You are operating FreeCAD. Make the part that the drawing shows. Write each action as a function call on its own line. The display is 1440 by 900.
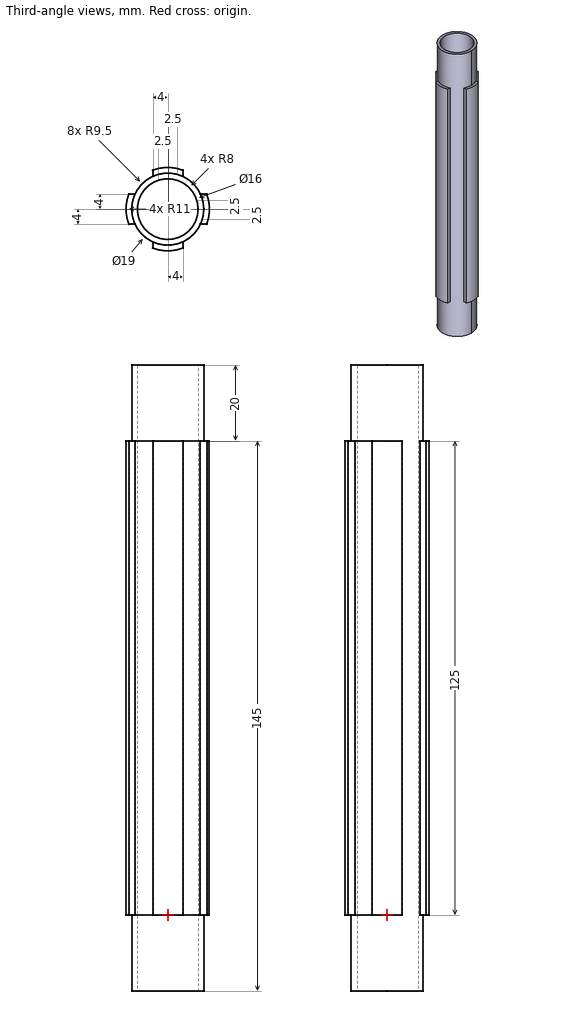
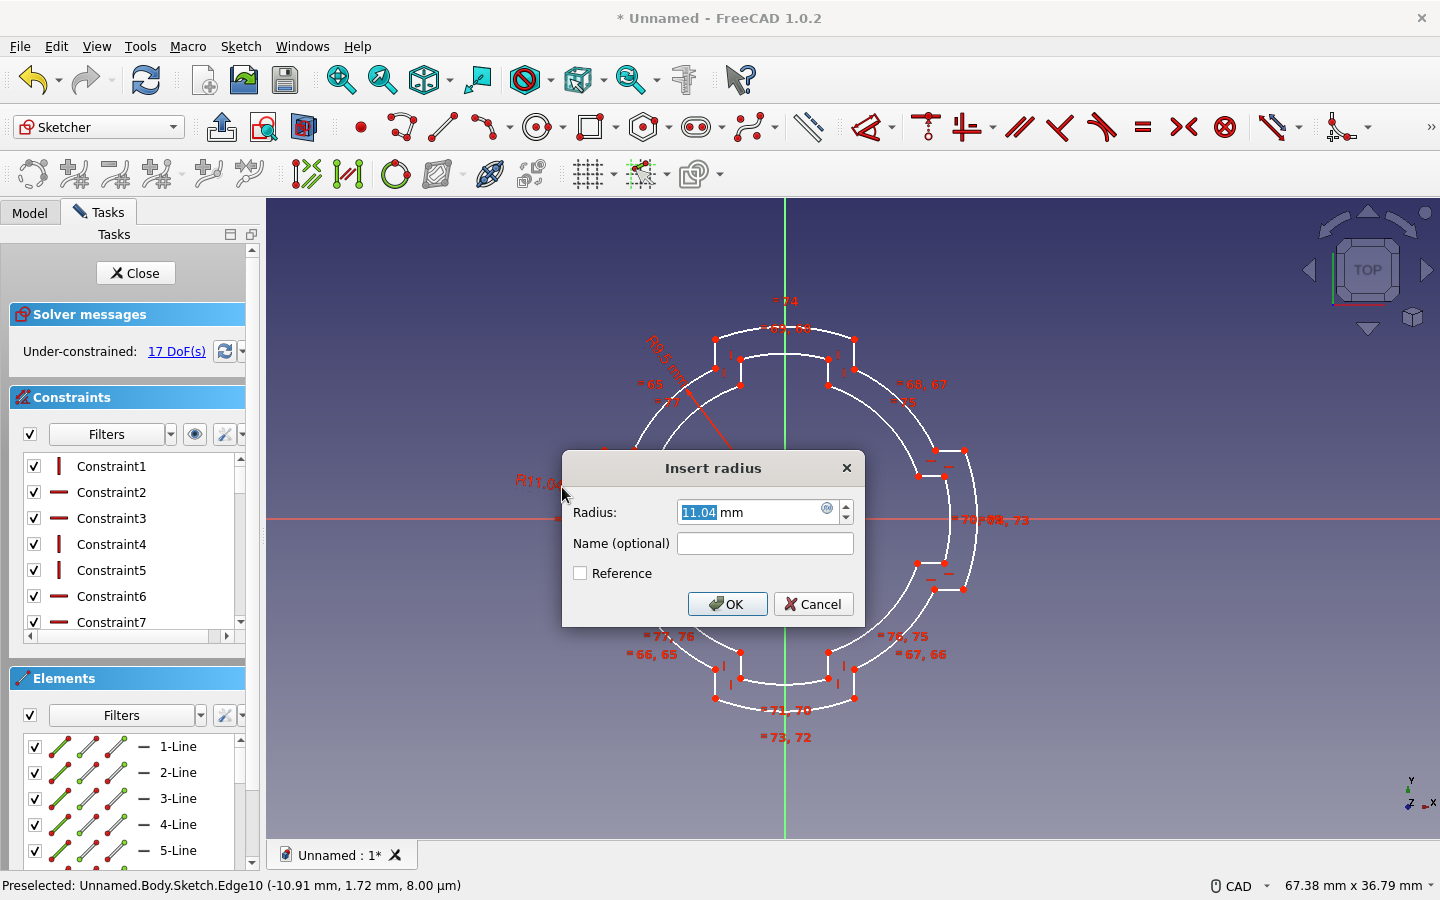
text(11)
key(Return)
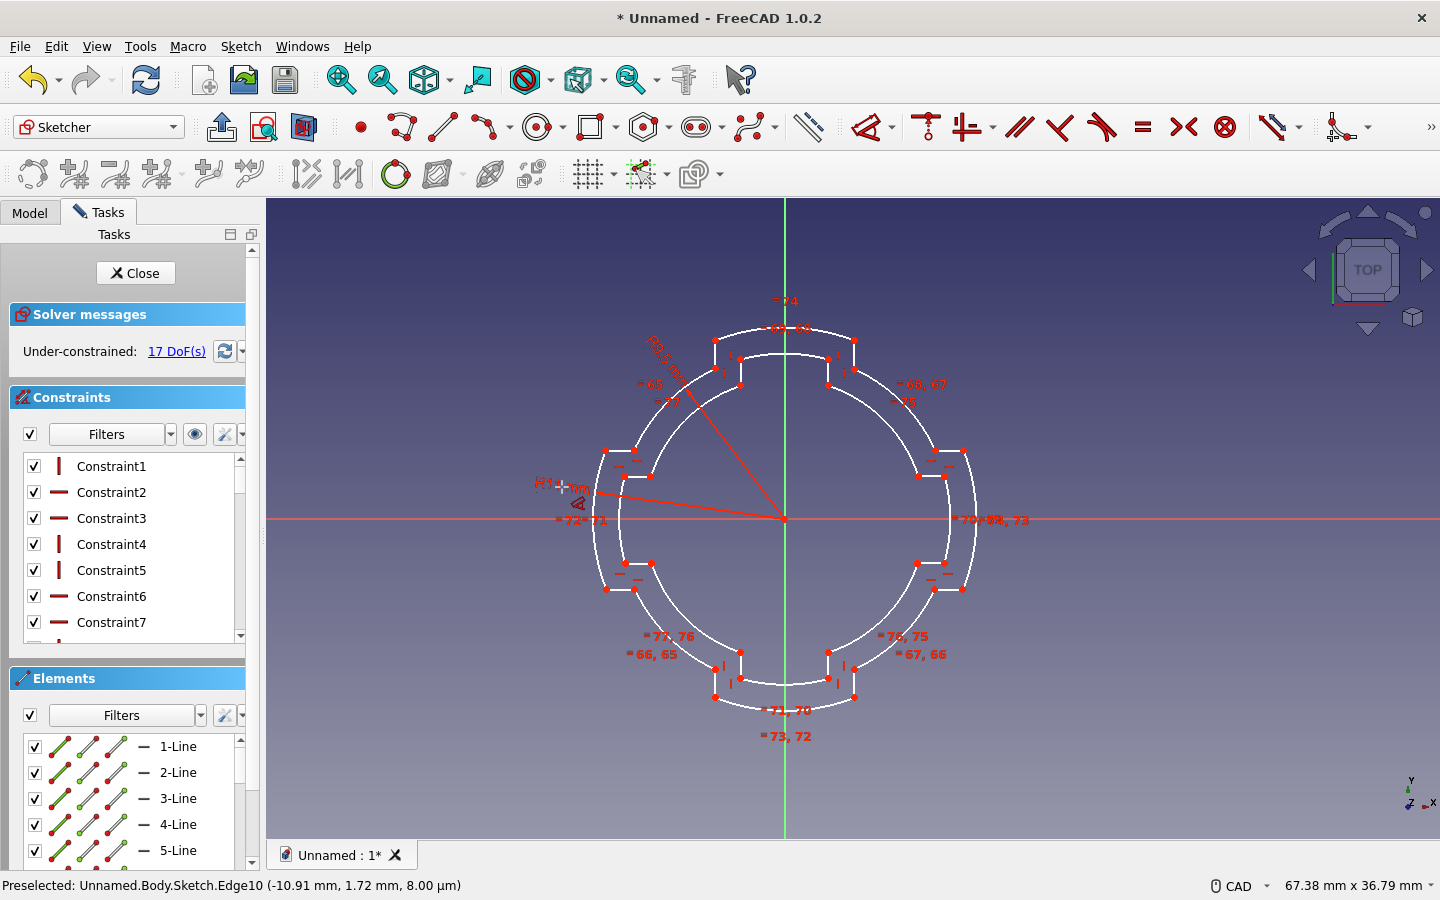
click(901, 440)
click(946, 409)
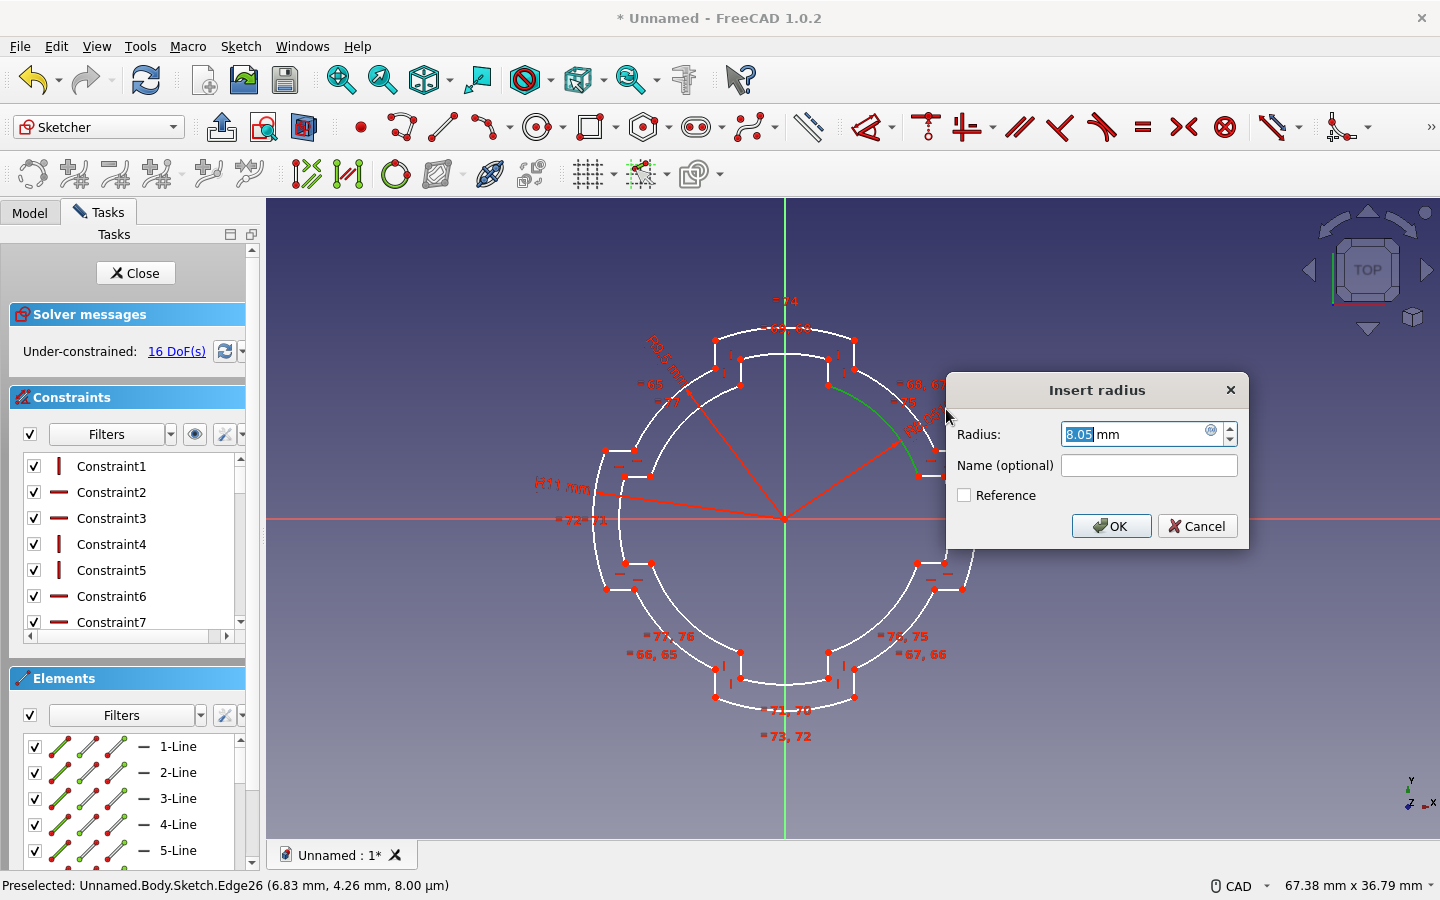
text(8)
key(Return)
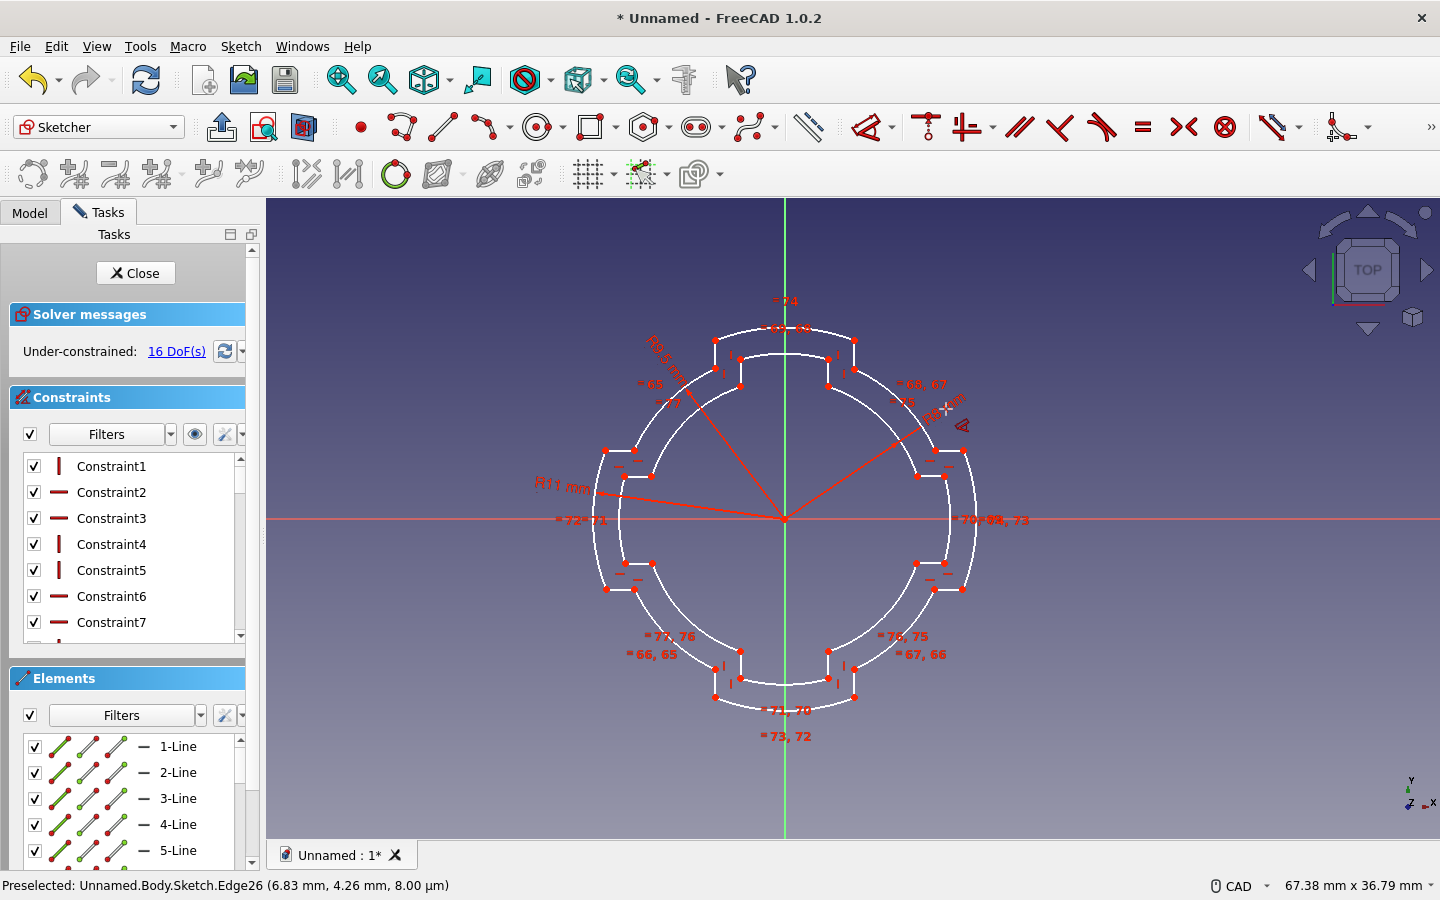
click(715, 341)
click(750, 307)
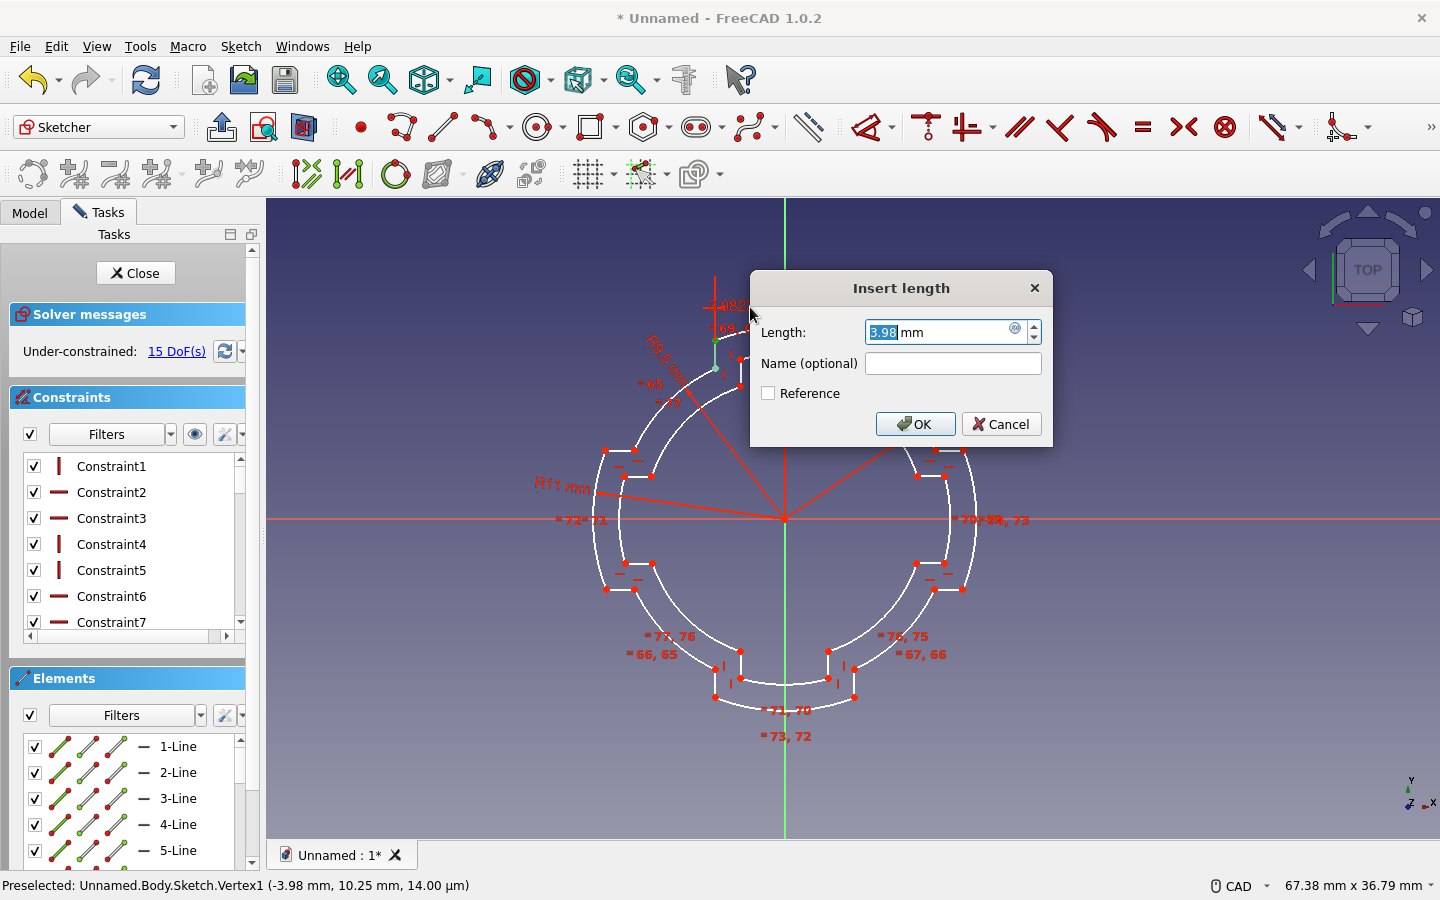
text(4)
key(Return)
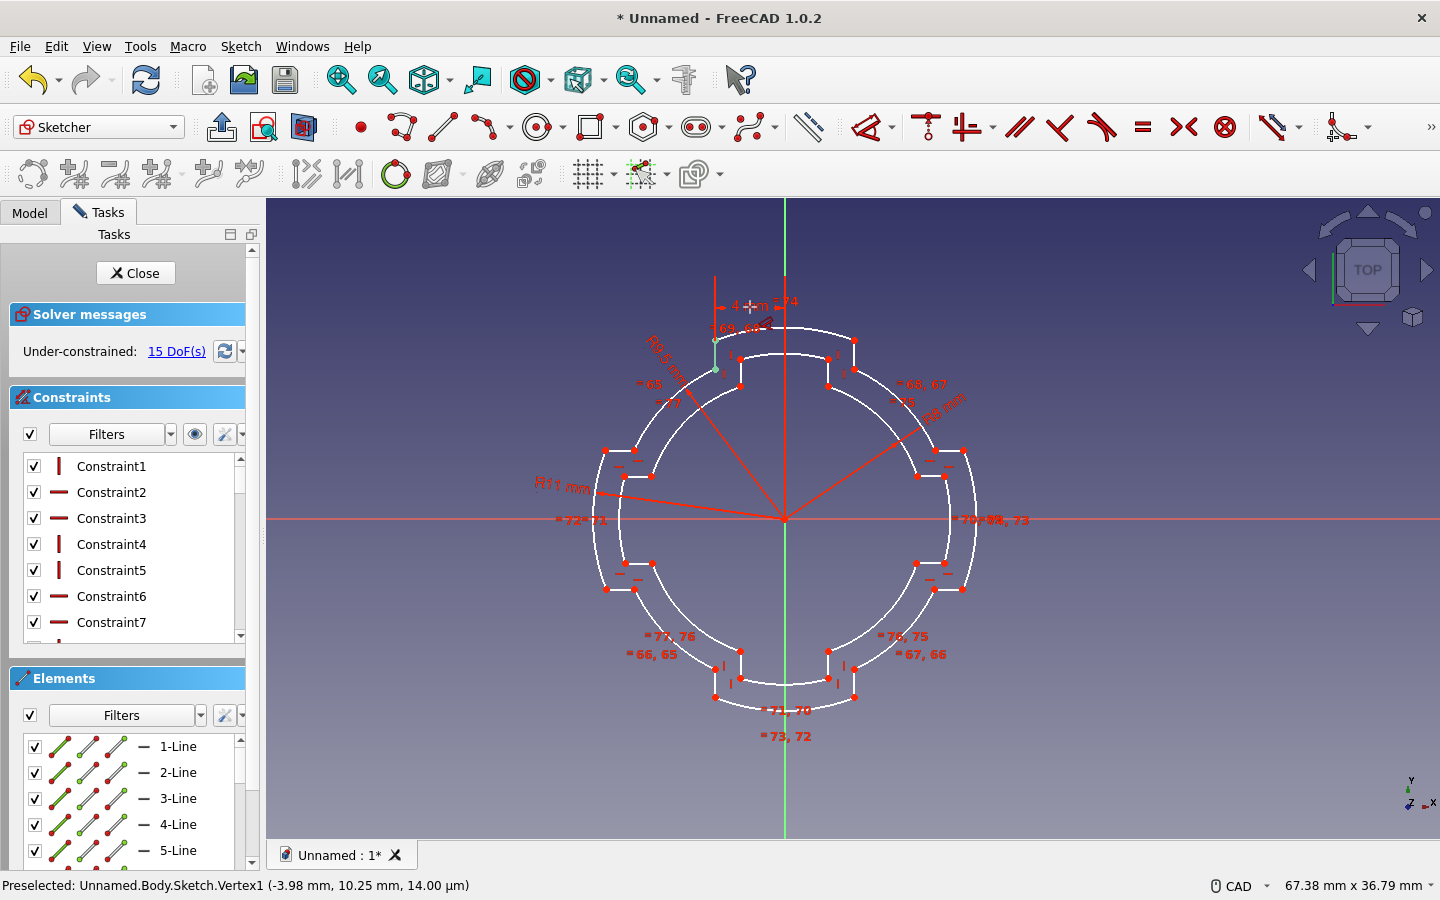
click(634, 451)
click(819, 485)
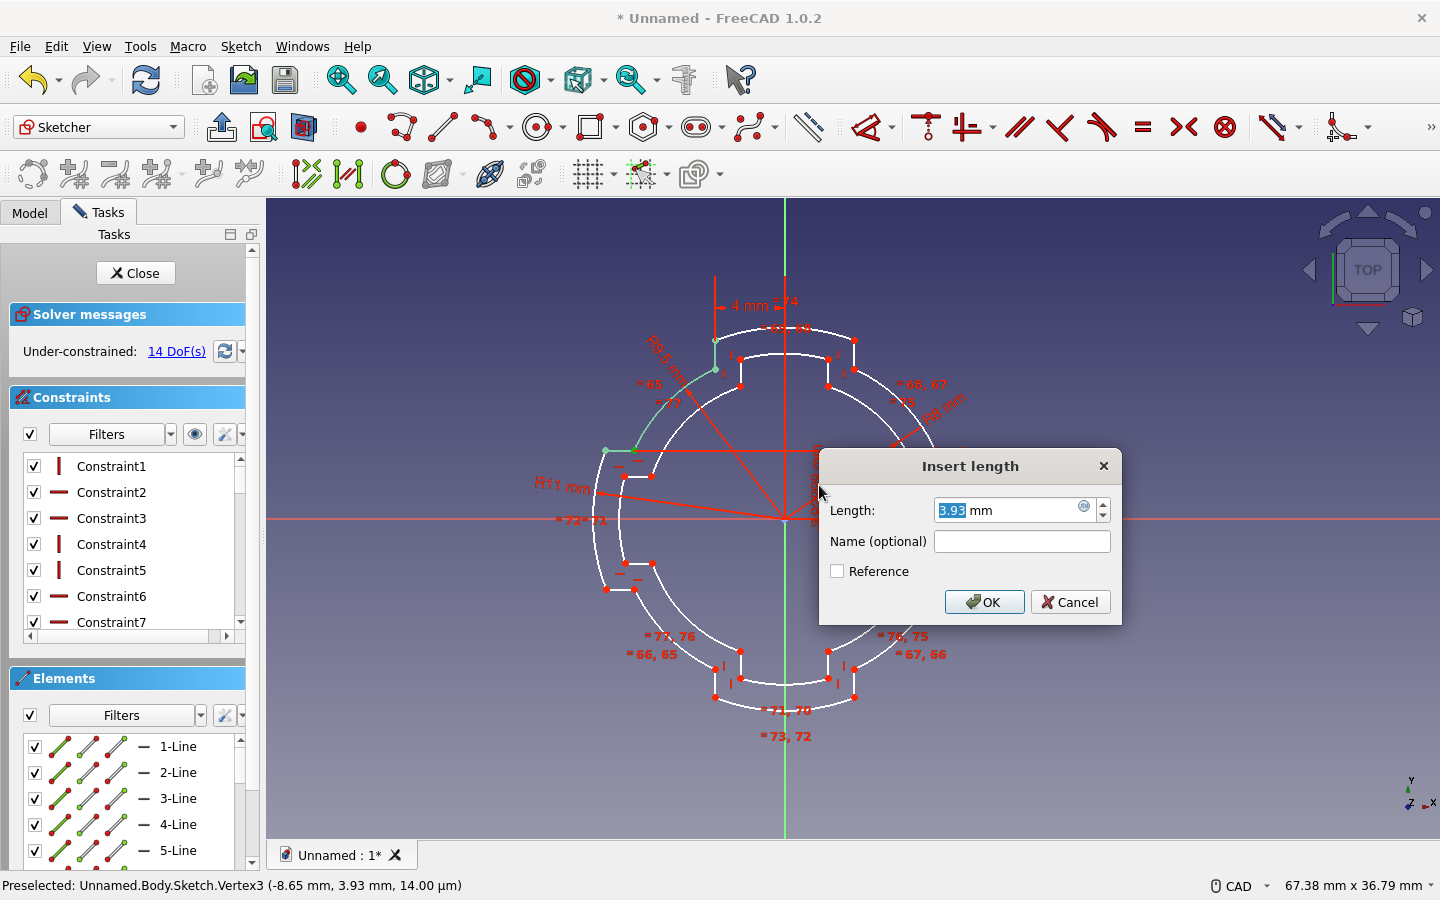
text(4)
key(Return)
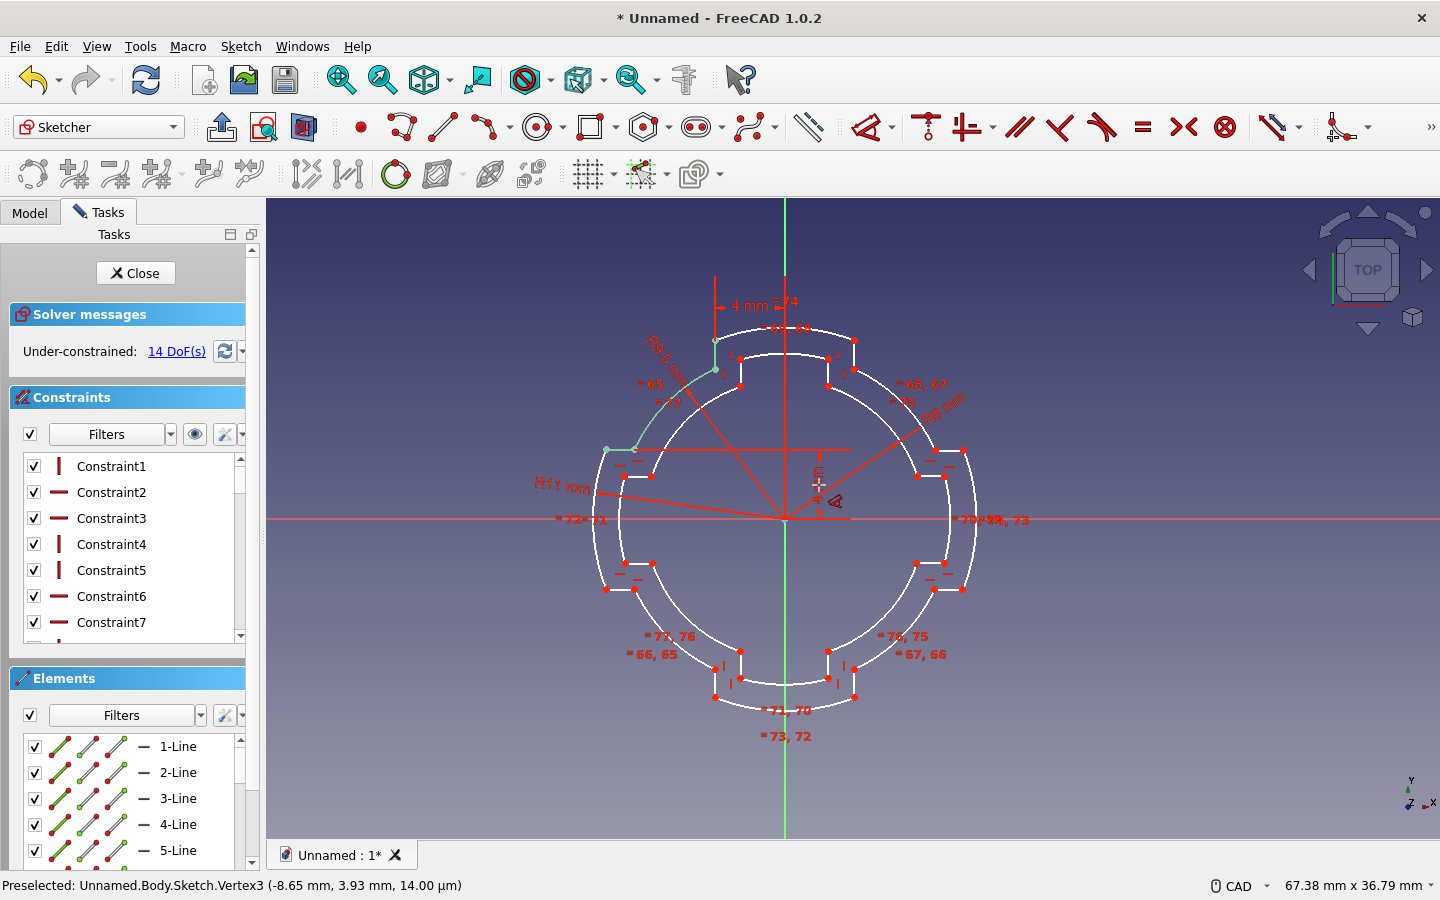
click(607, 590)
click(573, 555)